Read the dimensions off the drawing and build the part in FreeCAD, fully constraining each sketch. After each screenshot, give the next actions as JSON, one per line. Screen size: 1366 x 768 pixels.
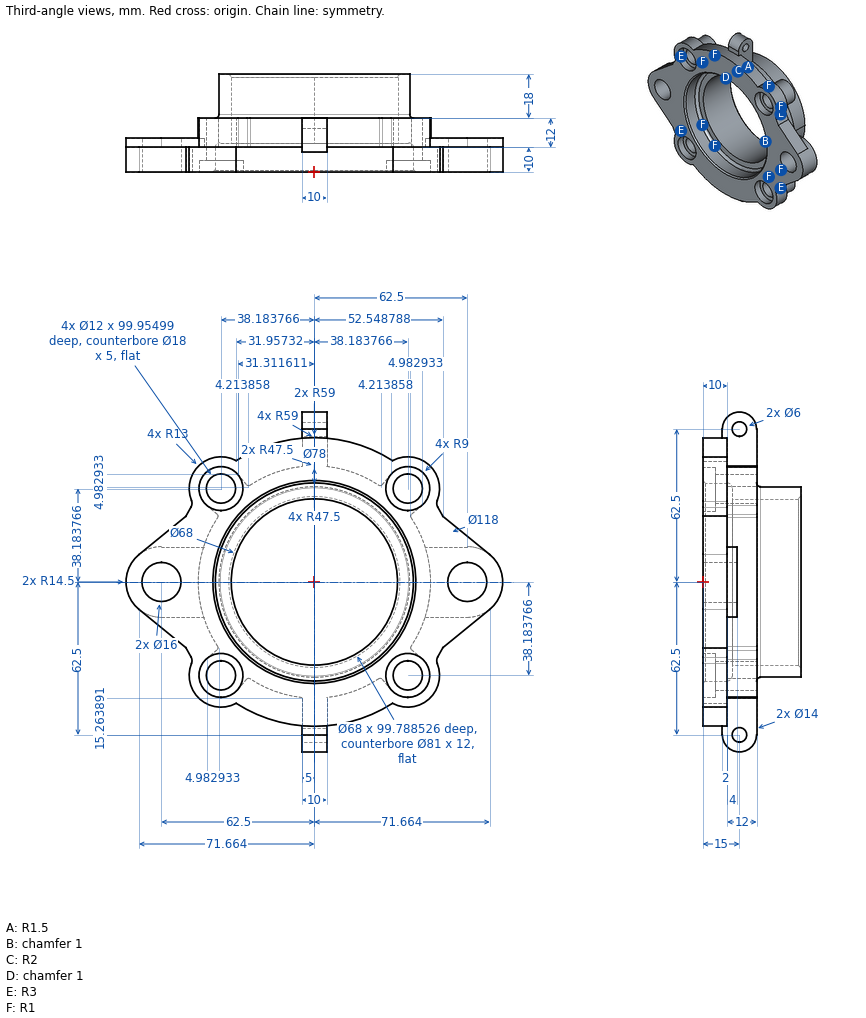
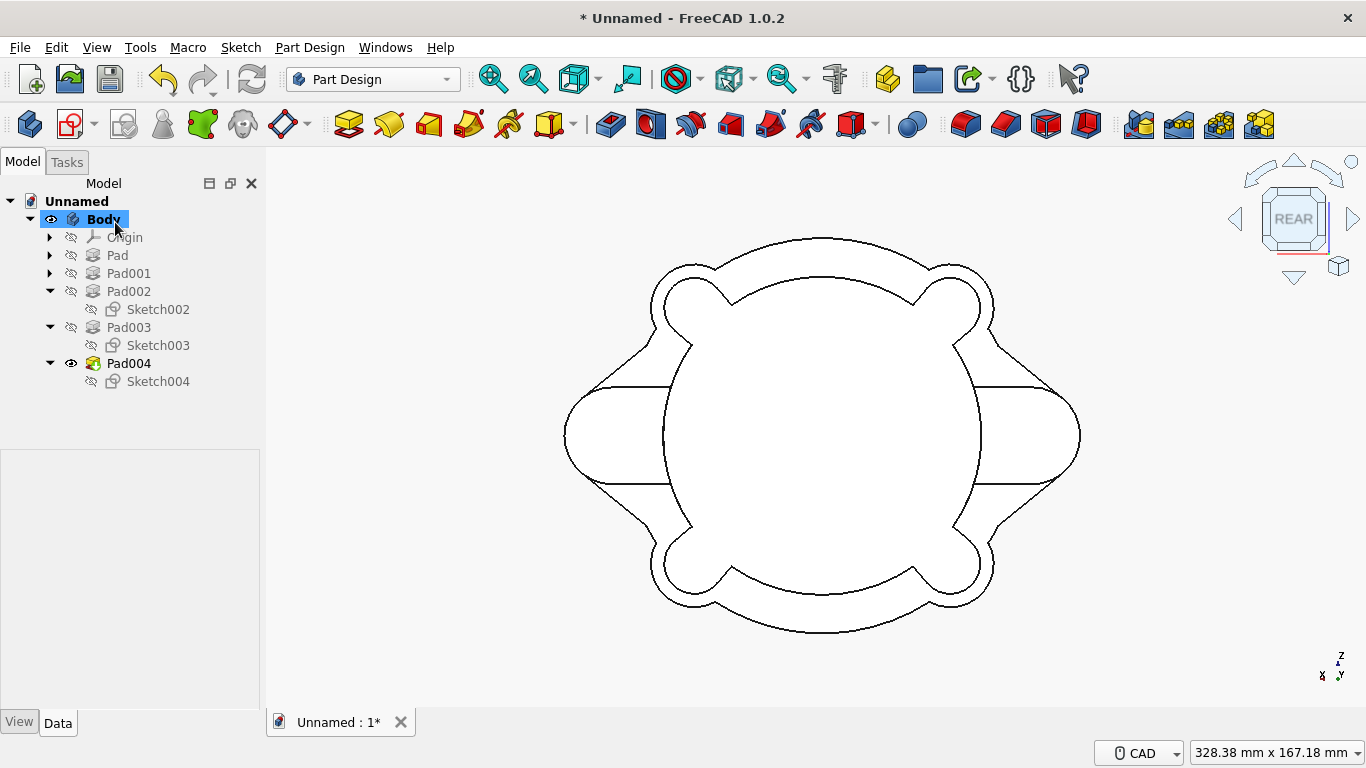
{"action": "left_click", "coordinate": [822, 435]}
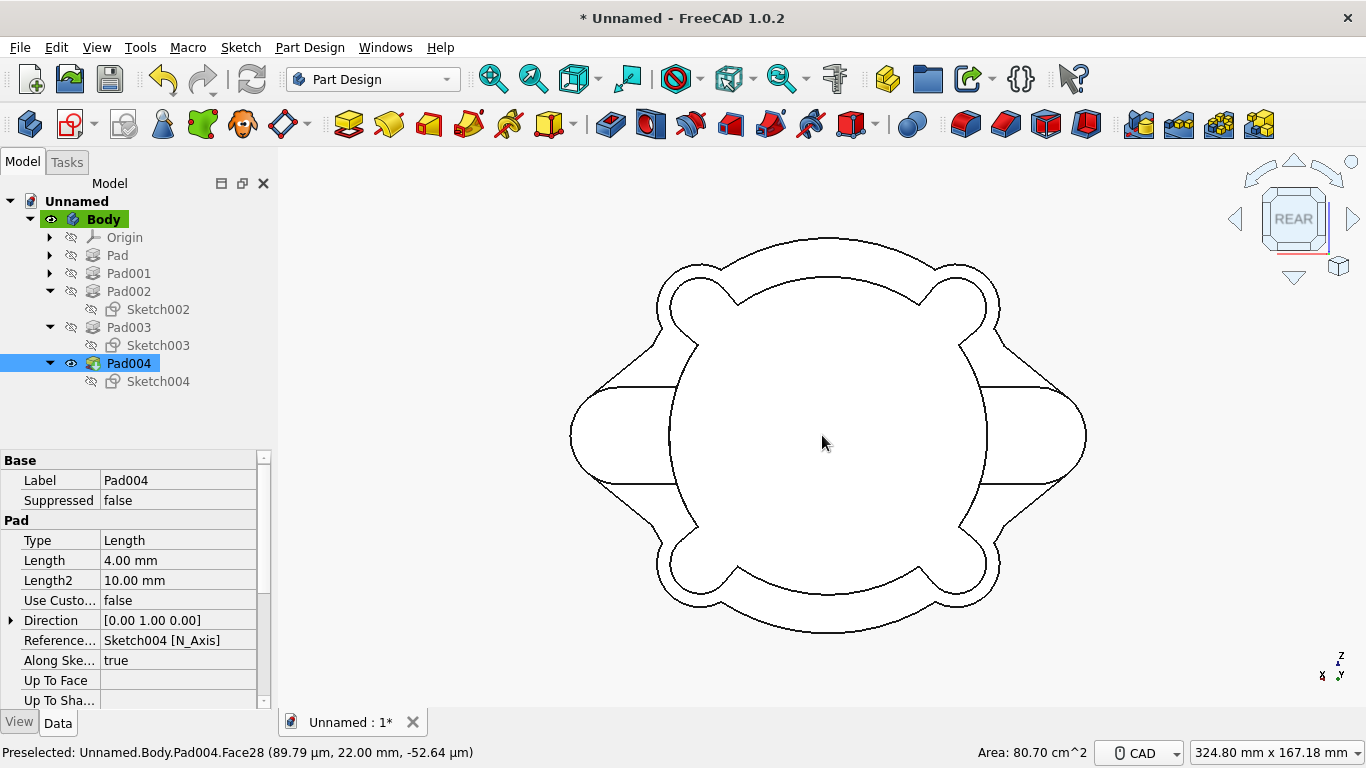
{"action": "left_click", "coordinate": [70, 124]}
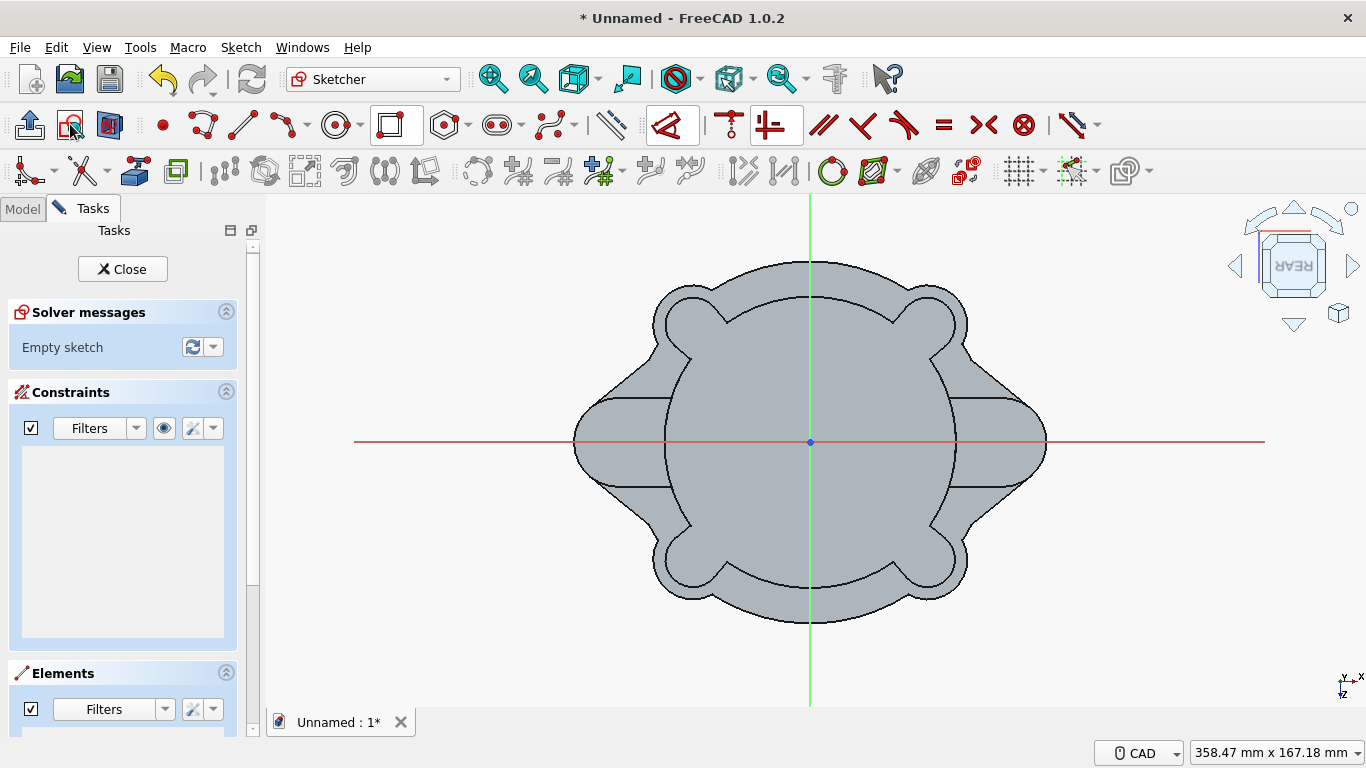
{"action": "left_click", "coordinate": [336, 126]}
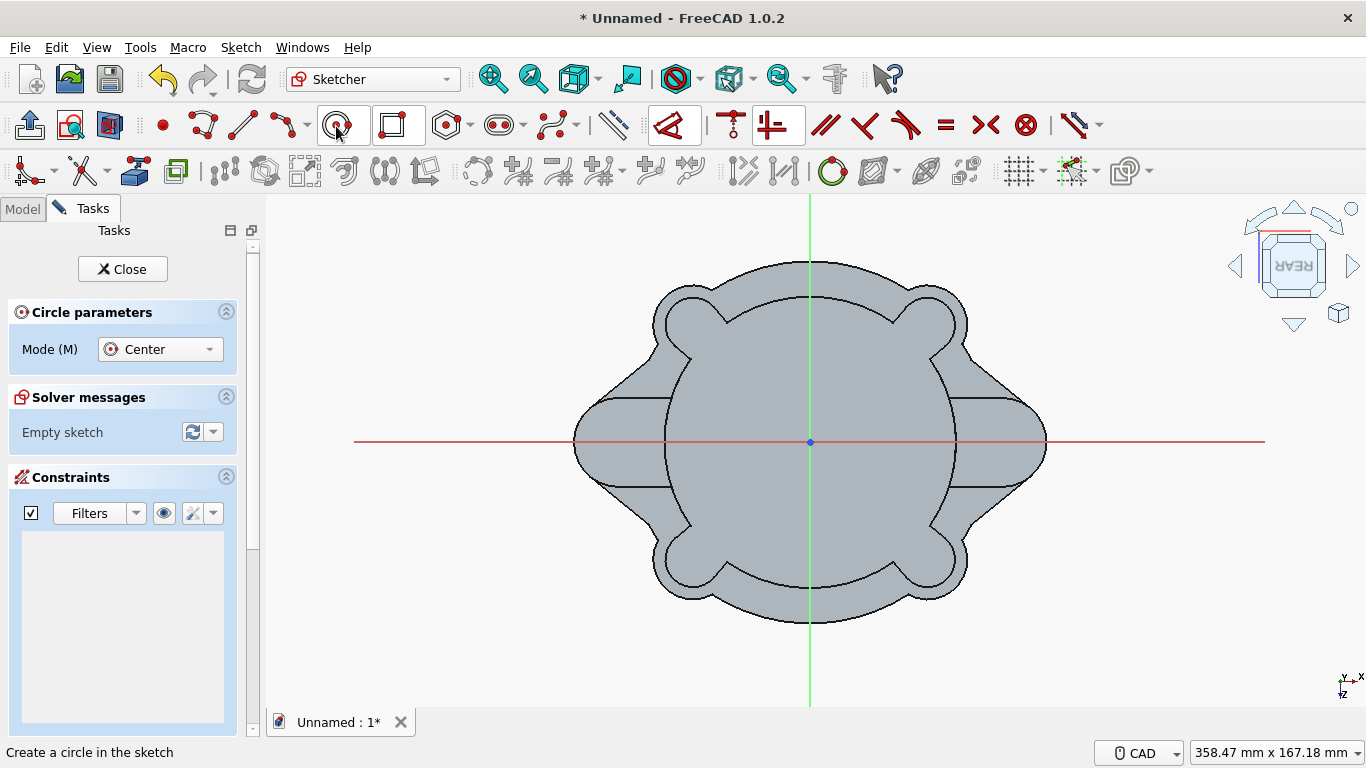
{"action": "left_click", "coordinate": [810, 442]}
{"action": "left_click", "coordinate": [895, 358]}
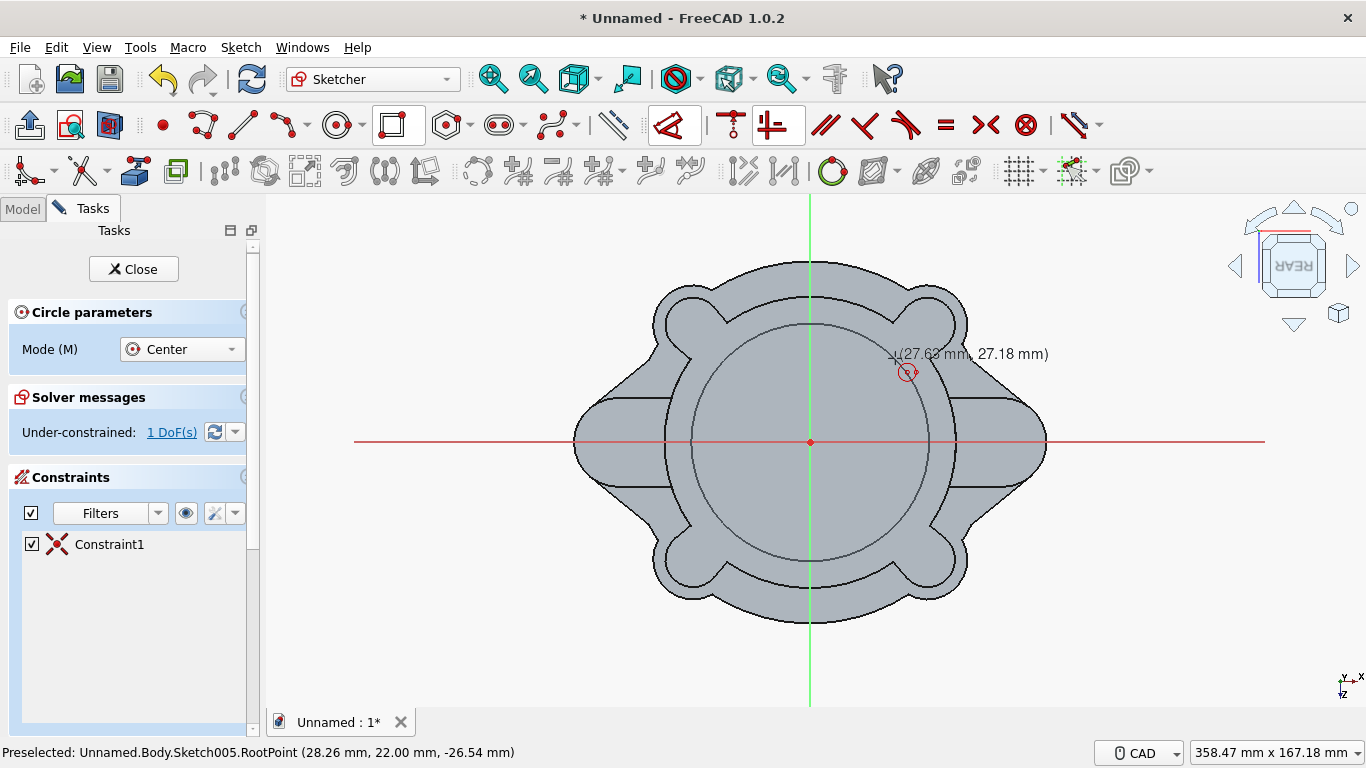
{"action": "left_click", "coordinate": [810, 442]}
{"action": "left_click", "coordinate": [884, 369]}
{"action": "key", "text": "Escape"}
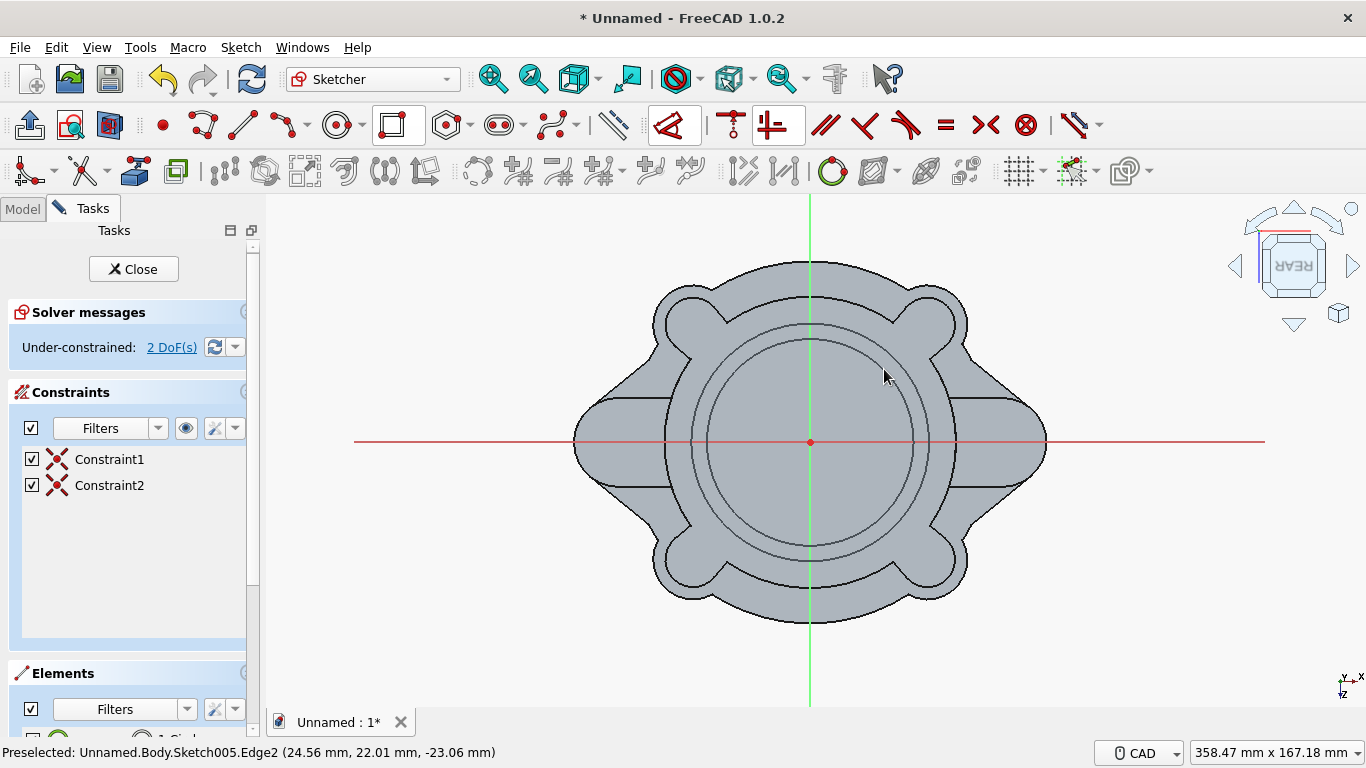
{"action": "left_click", "coordinate": [894, 358]}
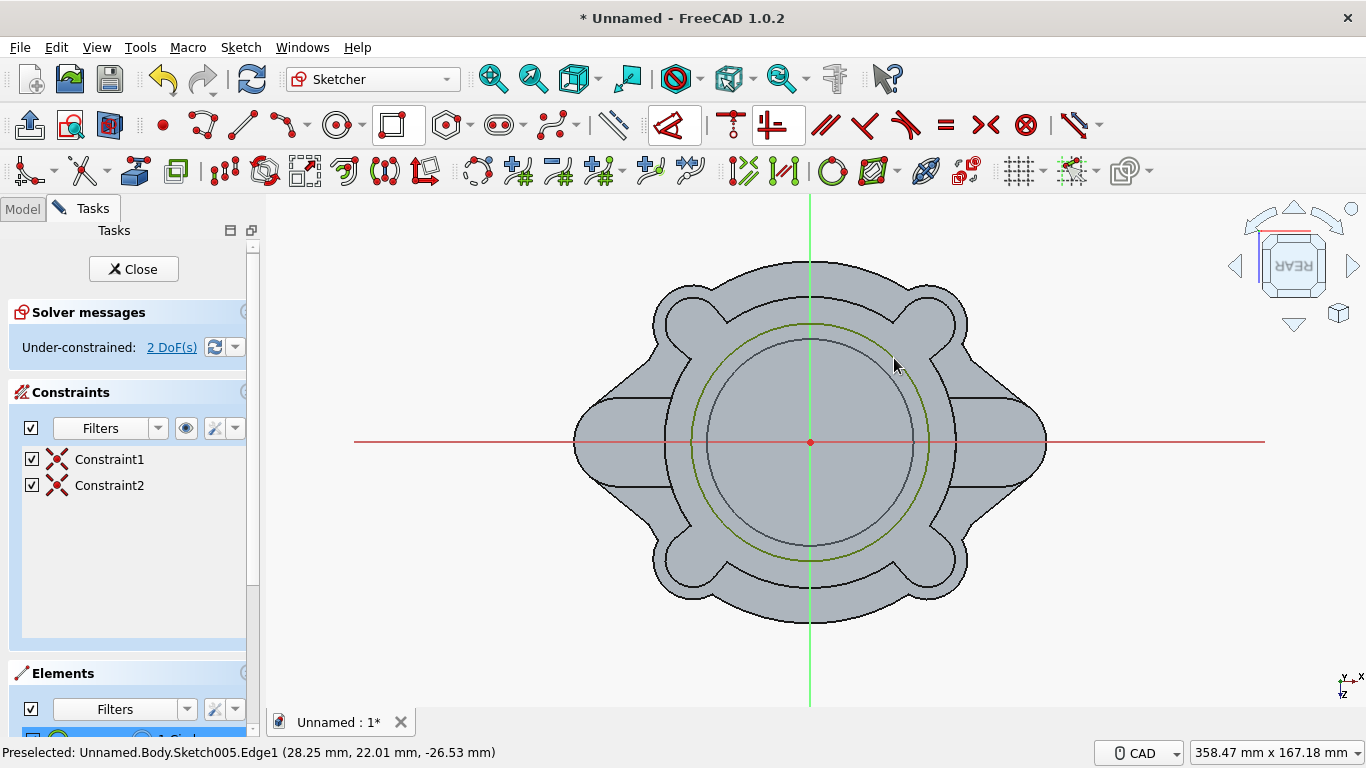
{"action": "key", "text": "k o"}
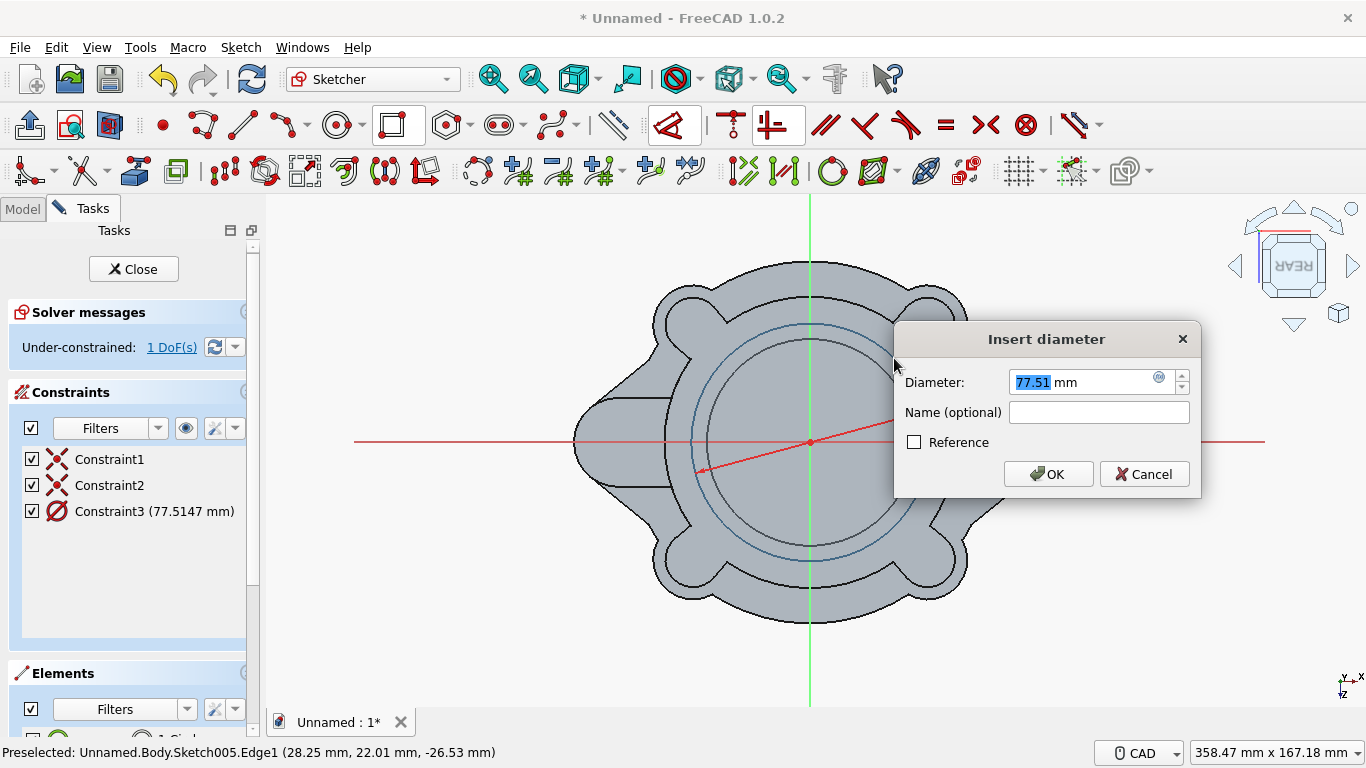
{"action": "type", "text": "78"}
{"action": "key", "text": "Return"}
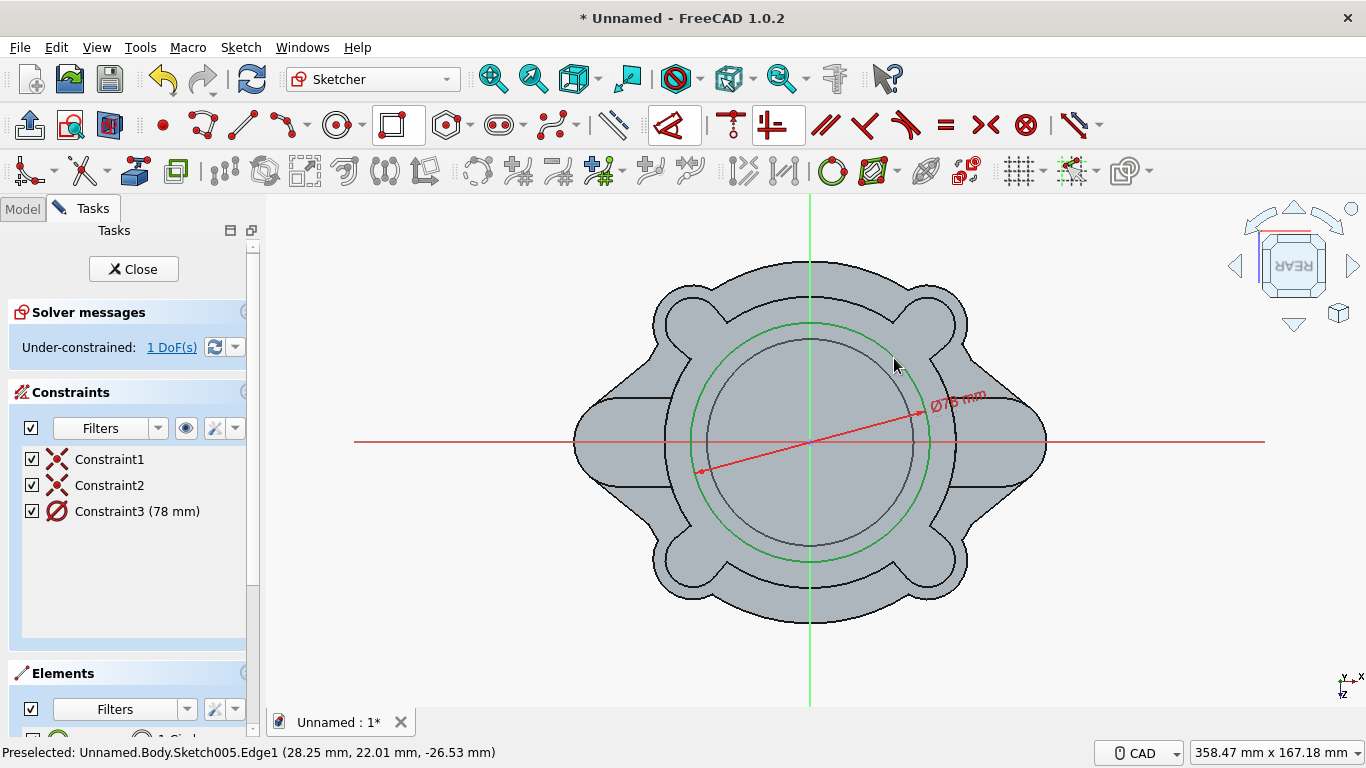
{"action": "left_click", "coordinate": [883, 369]}